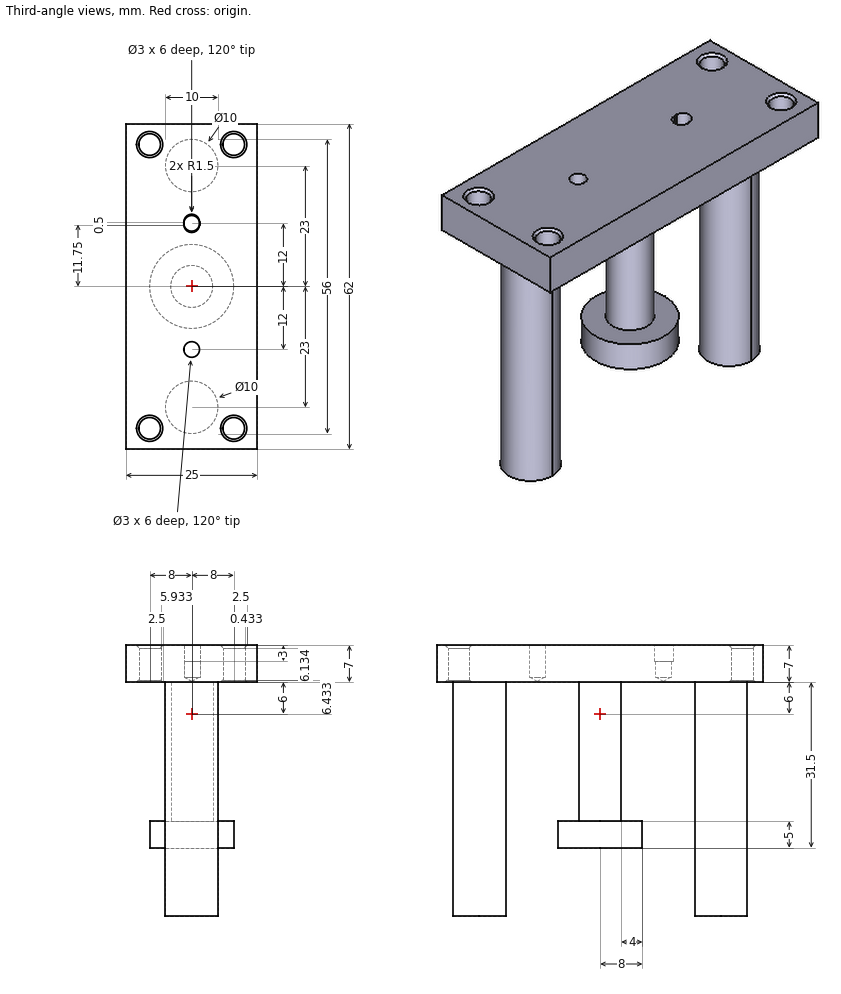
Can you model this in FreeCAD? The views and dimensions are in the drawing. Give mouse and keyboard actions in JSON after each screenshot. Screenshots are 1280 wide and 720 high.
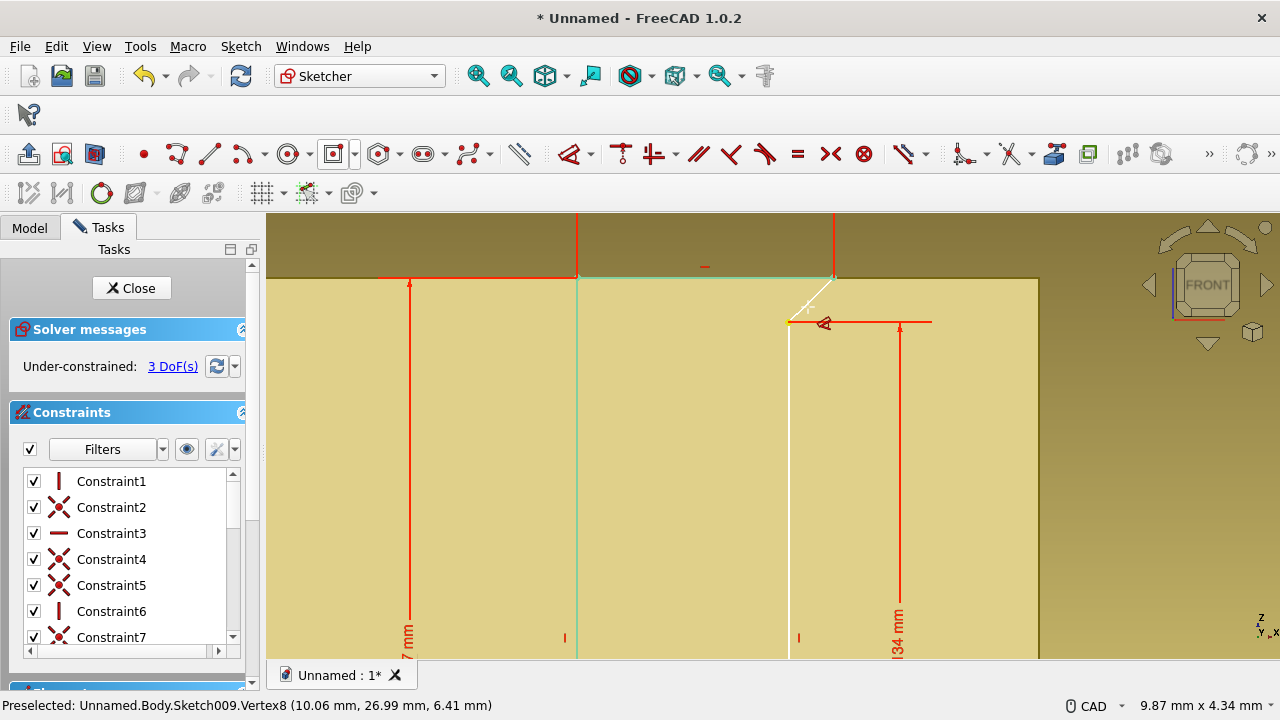
{"action": "left_click", "coordinate": [807, 305]}
{"action": "left_click", "coordinate": [811, 244]}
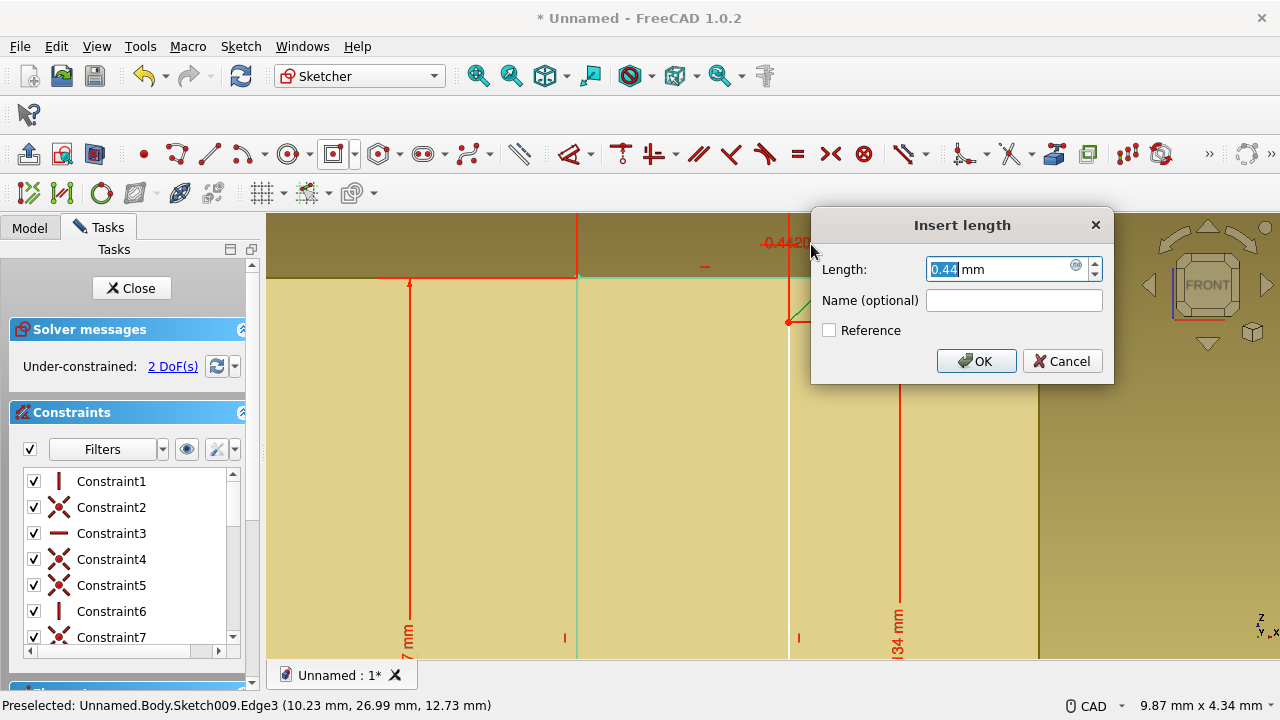
{"action": "type", "text": "0.433"}
{"action": "key", "text": "Return"}
{"action": "key", "text": "Escape"}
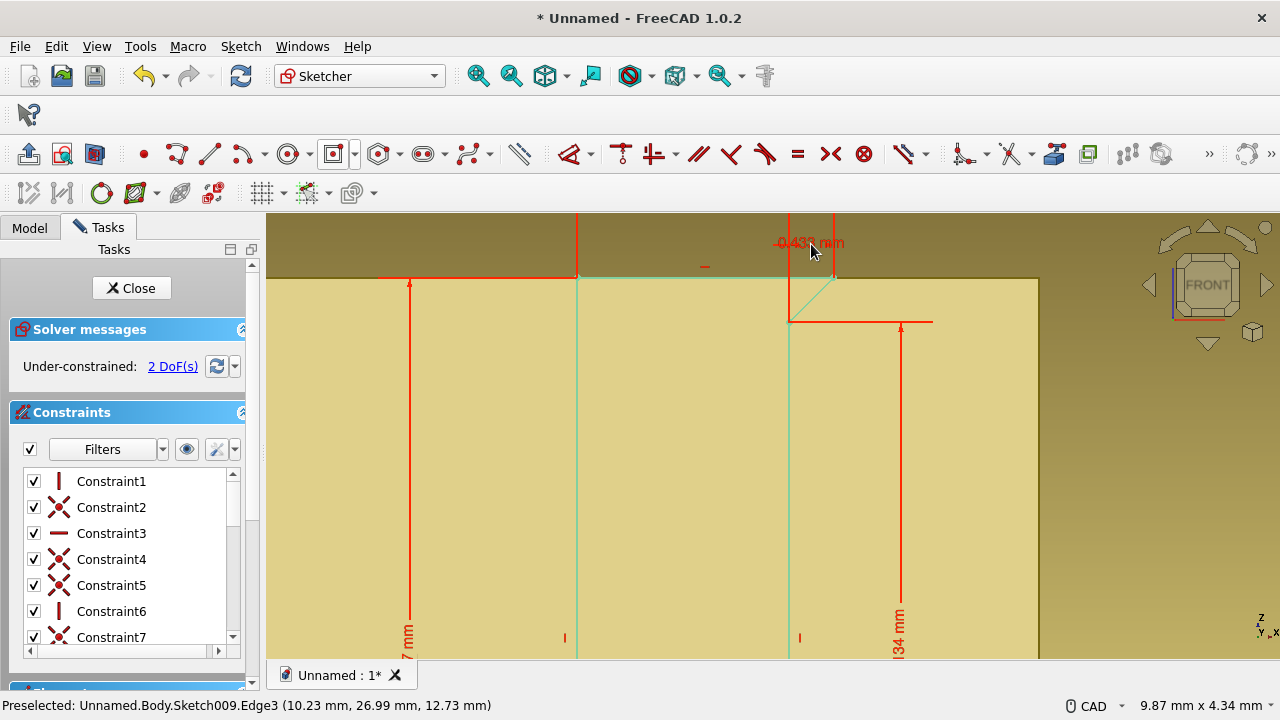
{"action": "left_click", "coordinate": [132, 288]}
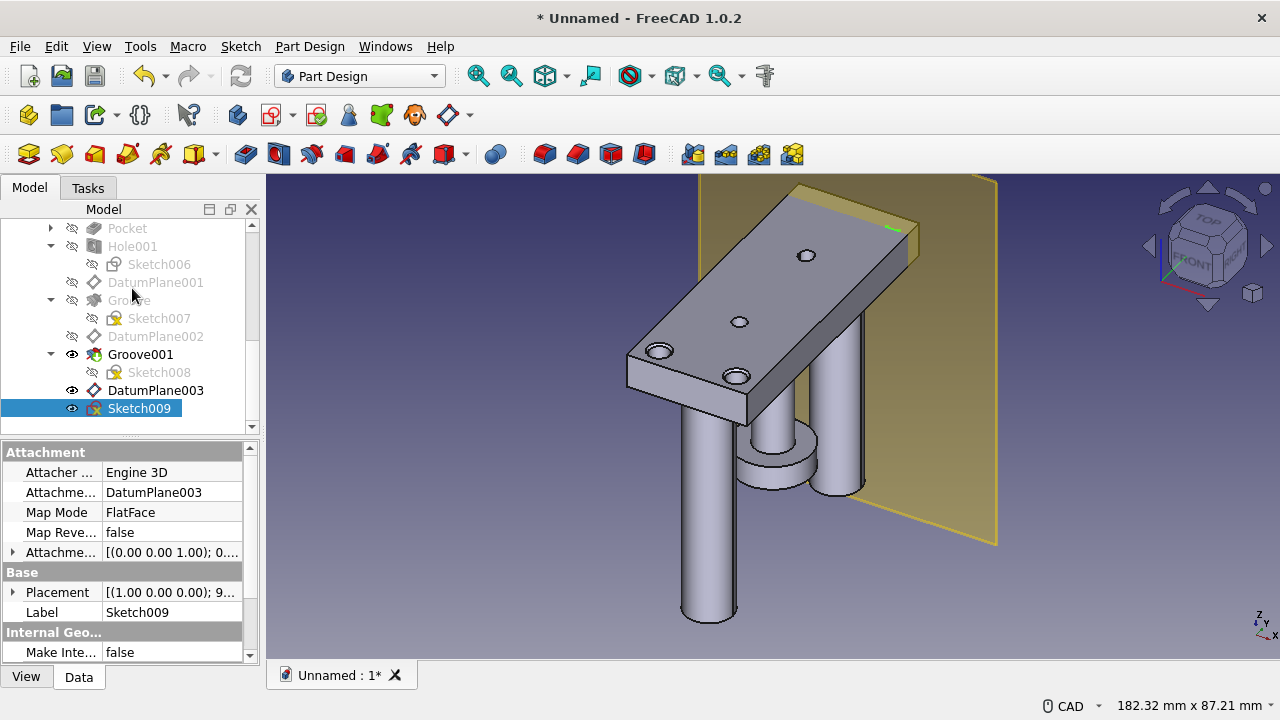
{"action": "left_click", "coordinate": [312, 154]}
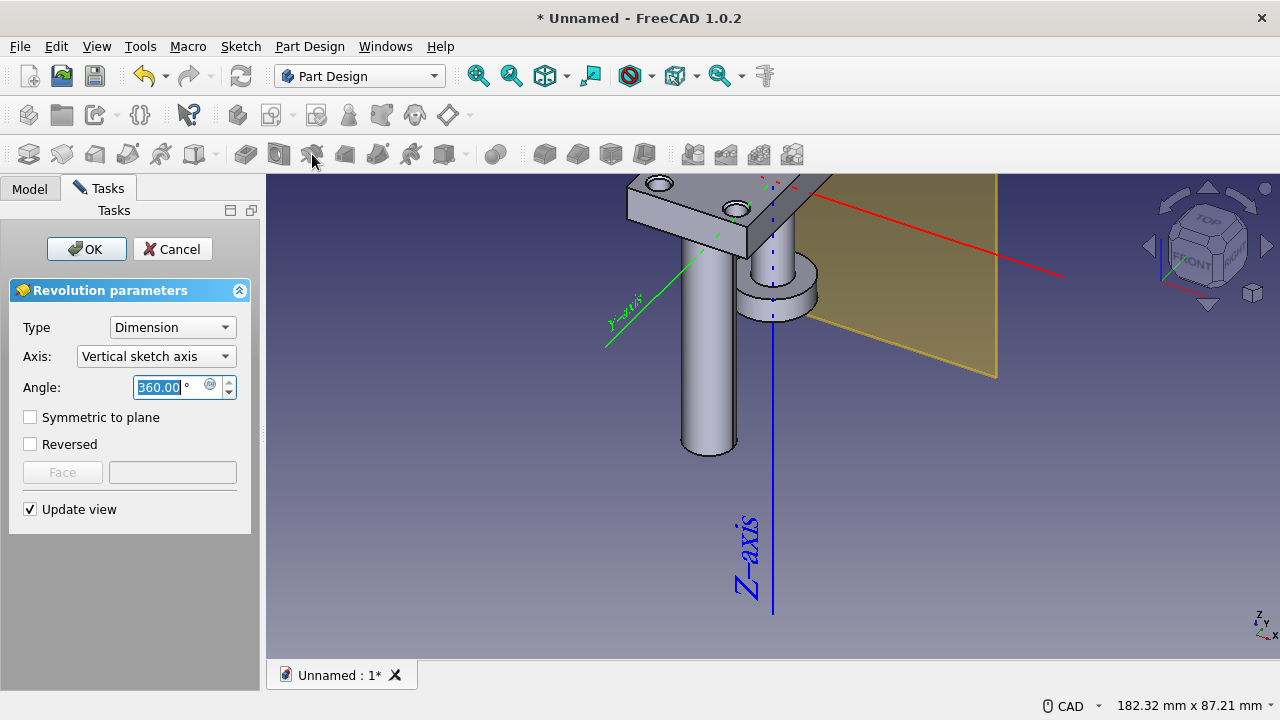
{"action": "left_click", "coordinate": [157, 356]}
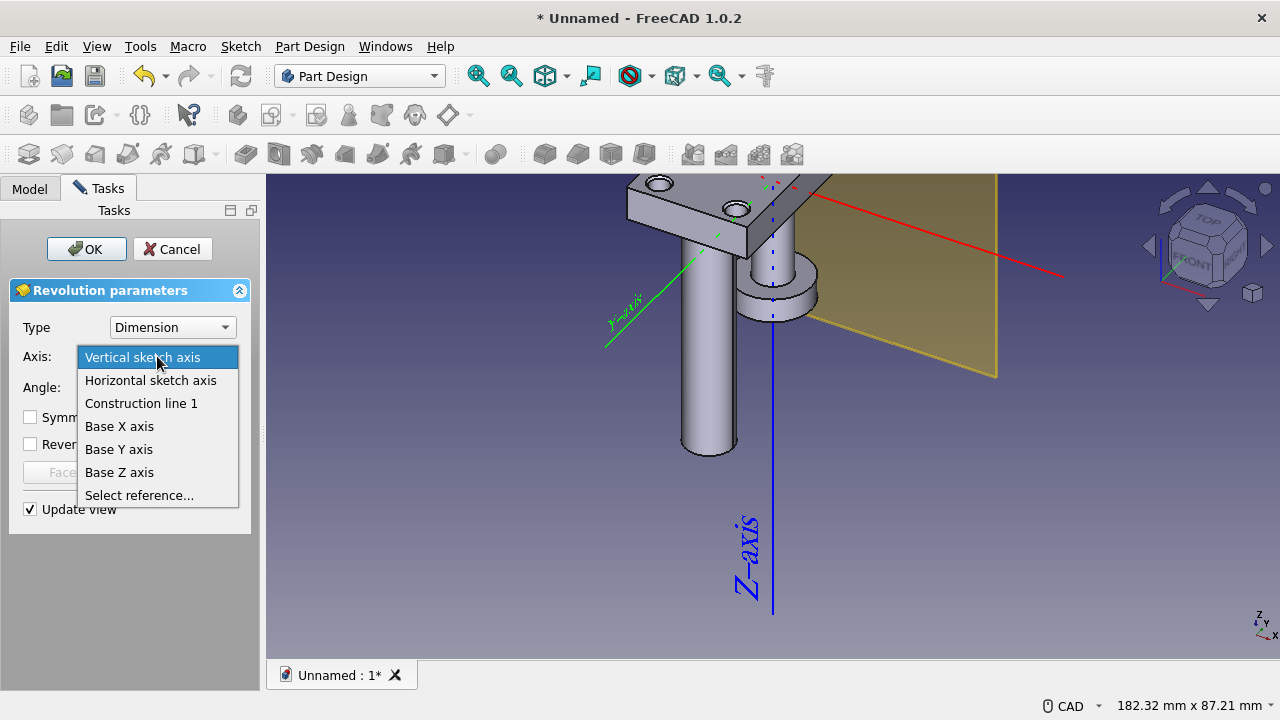
{"action": "left_click", "coordinate": [156, 404]}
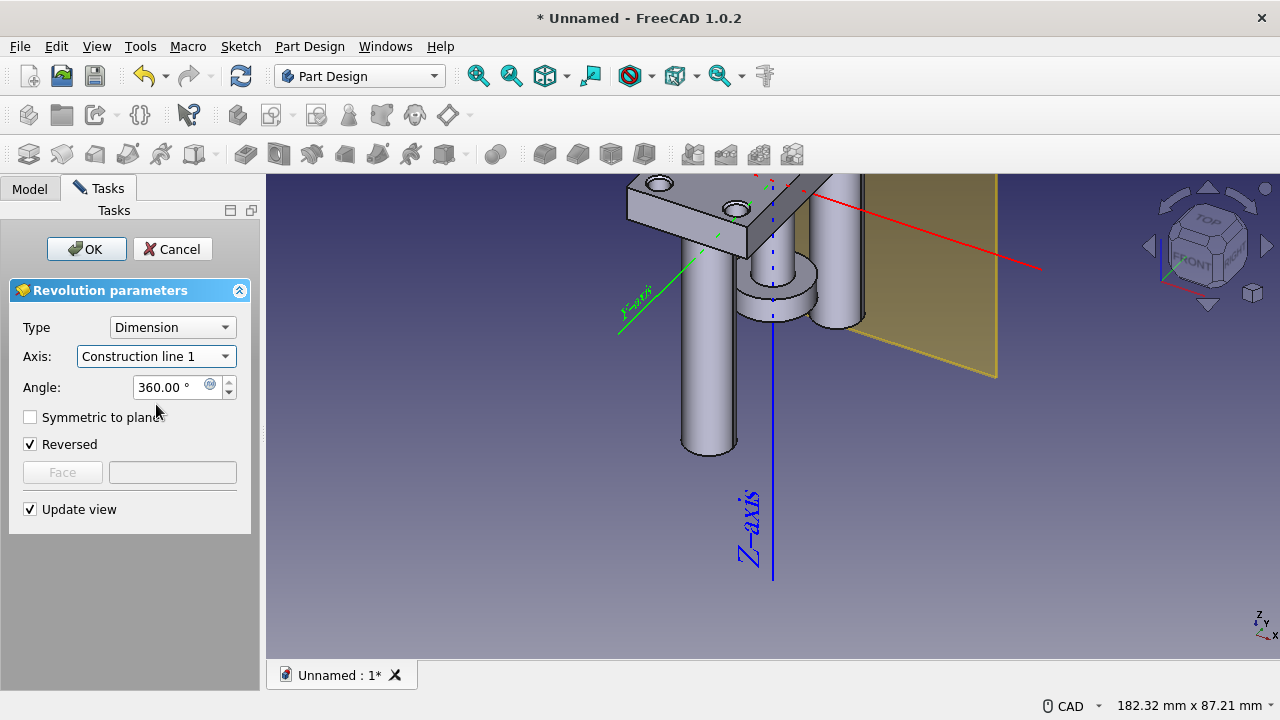
{"action": "left_click", "coordinate": [87, 249]}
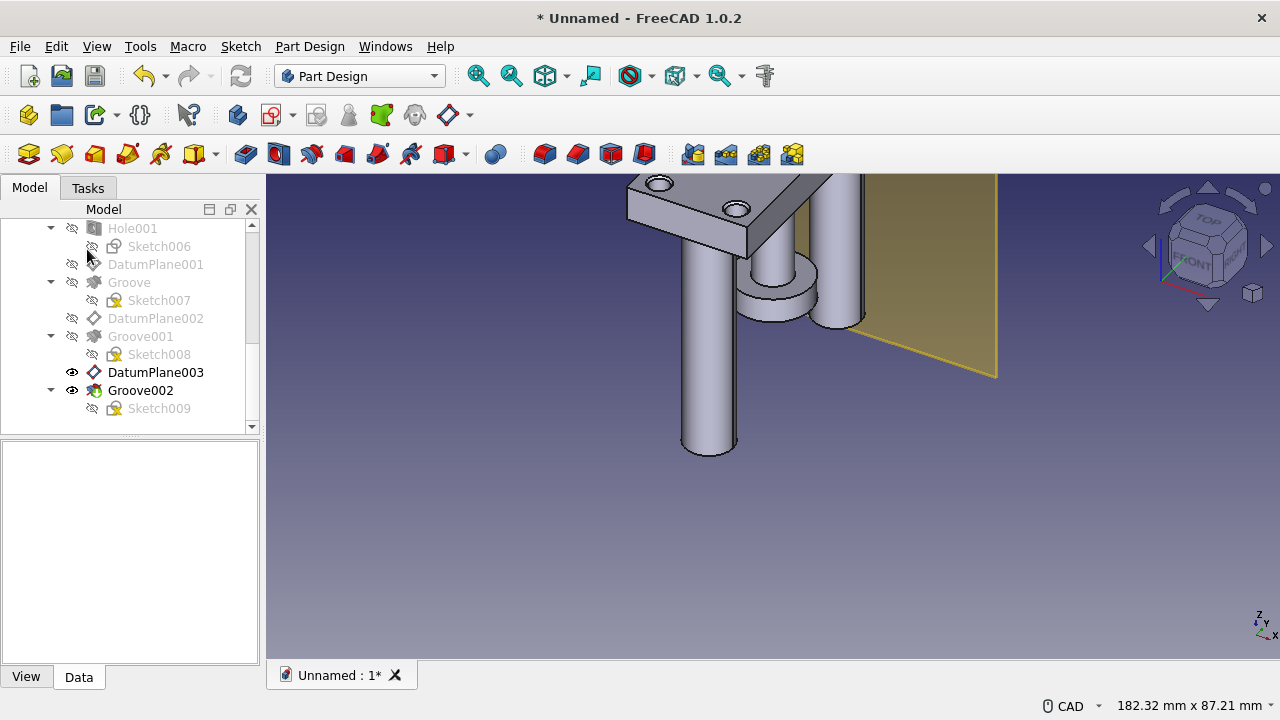
{"action": "left_click", "coordinate": [117, 372]}
{"action": "key", "text": "space"}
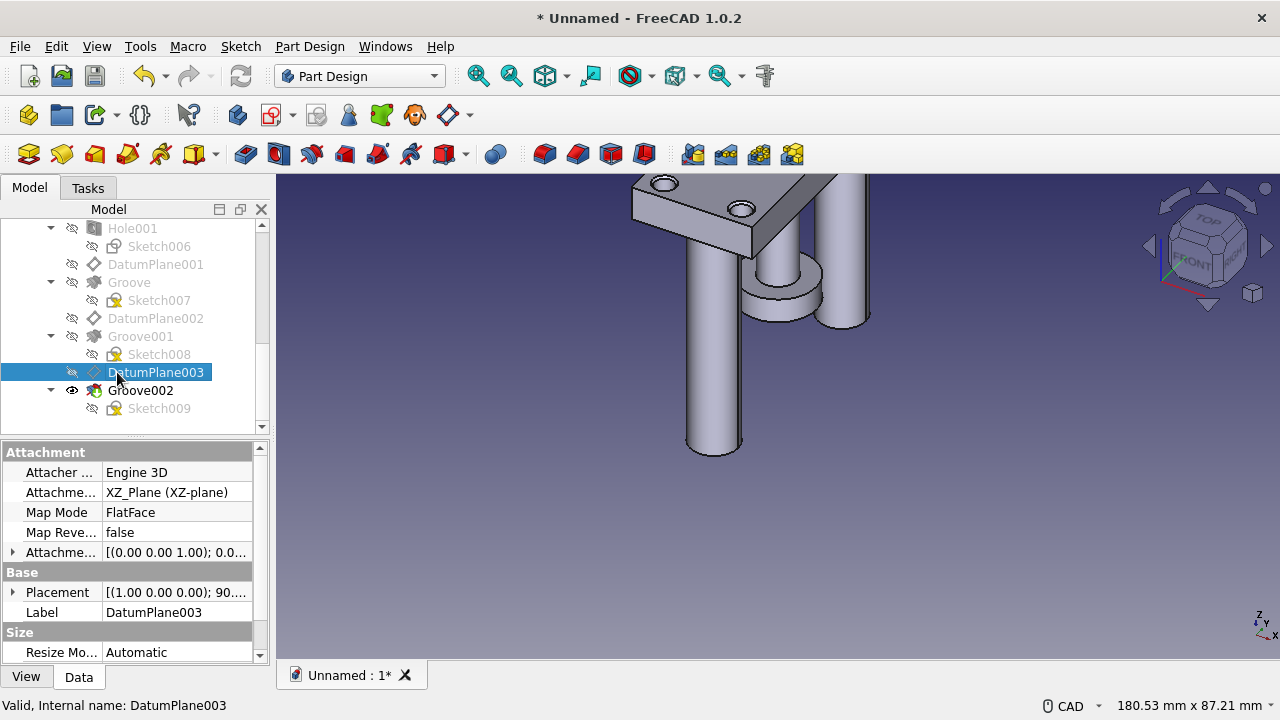
{"action": "left_click", "coordinate": [479, 76]}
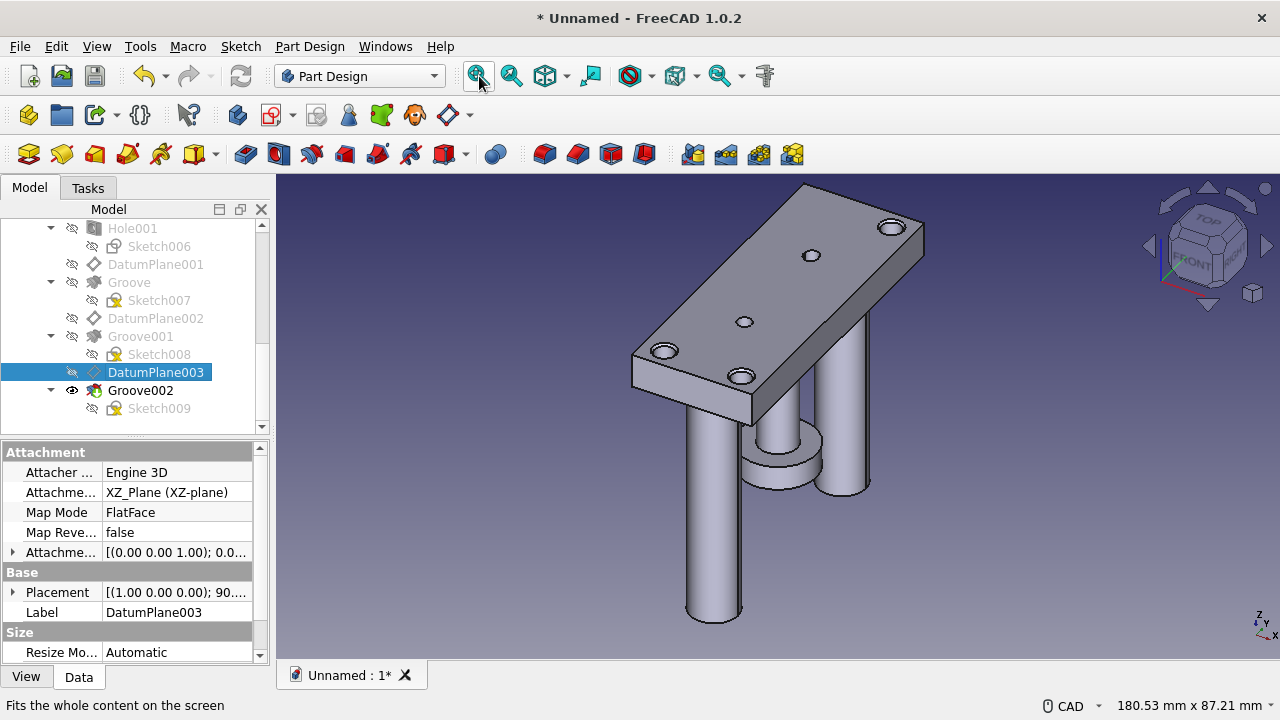
{"action": "scroll", "coordinate": [141, 314], "scroll_direction": "down", "scroll_amount": 3}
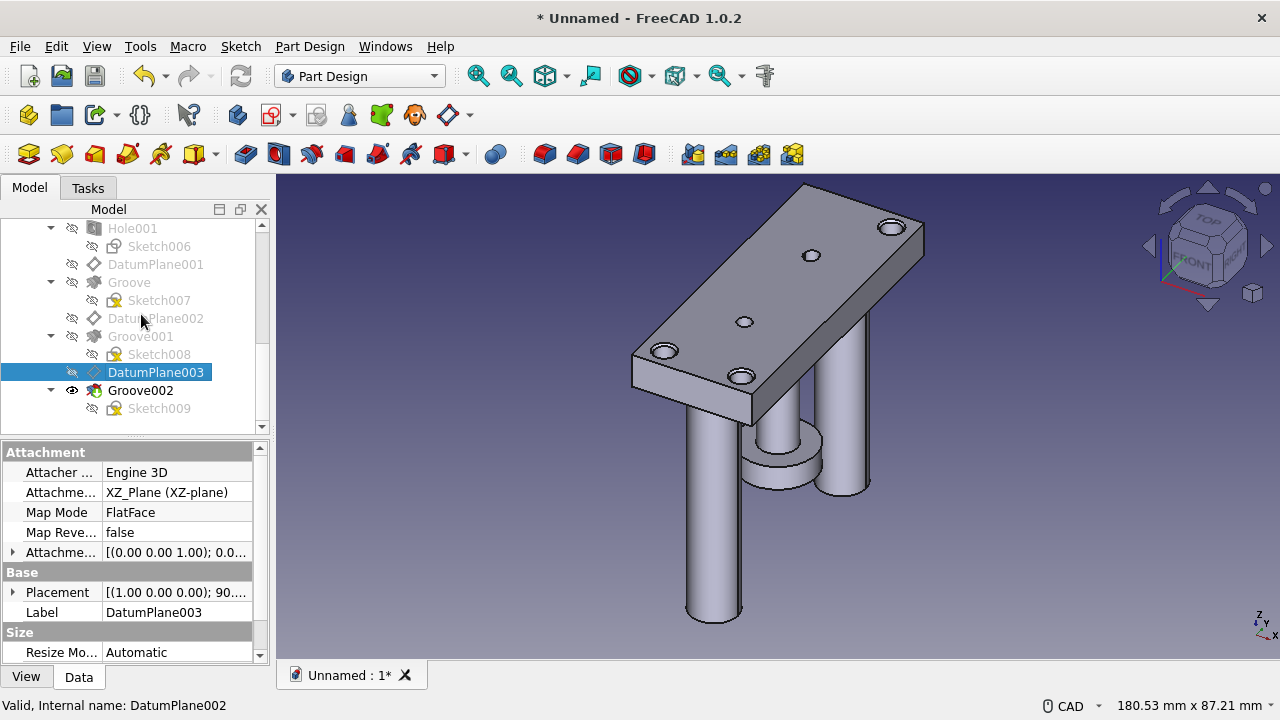
{"action": "scroll", "coordinate": [141, 314], "scroll_direction": "up", "scroll_amount": 15}